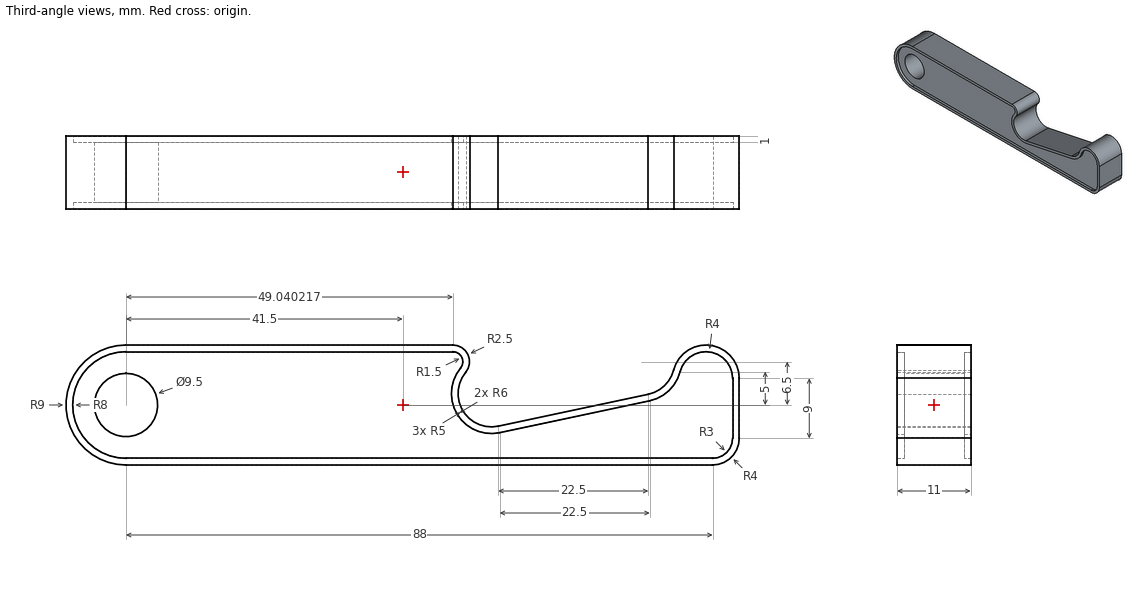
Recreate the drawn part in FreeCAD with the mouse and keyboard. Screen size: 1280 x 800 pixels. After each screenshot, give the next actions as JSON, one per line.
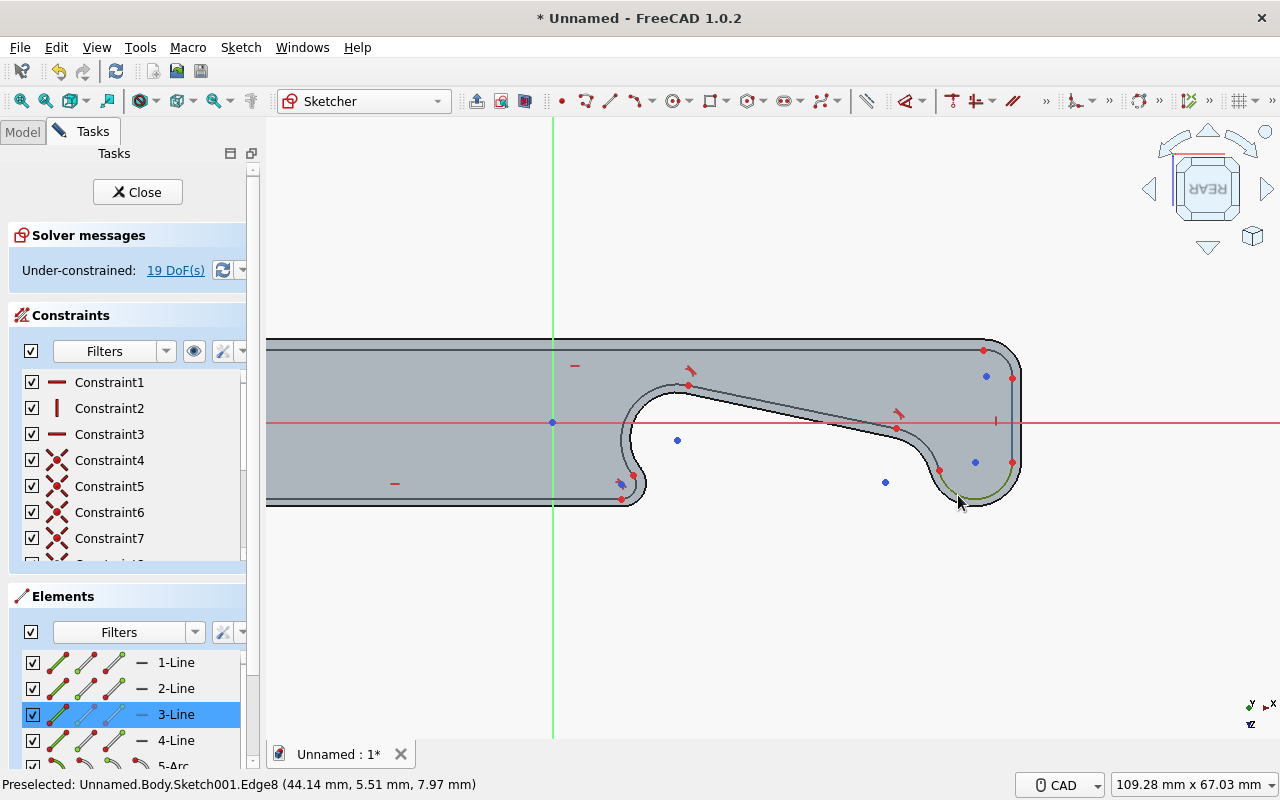
{"action": "key", "text": "t"}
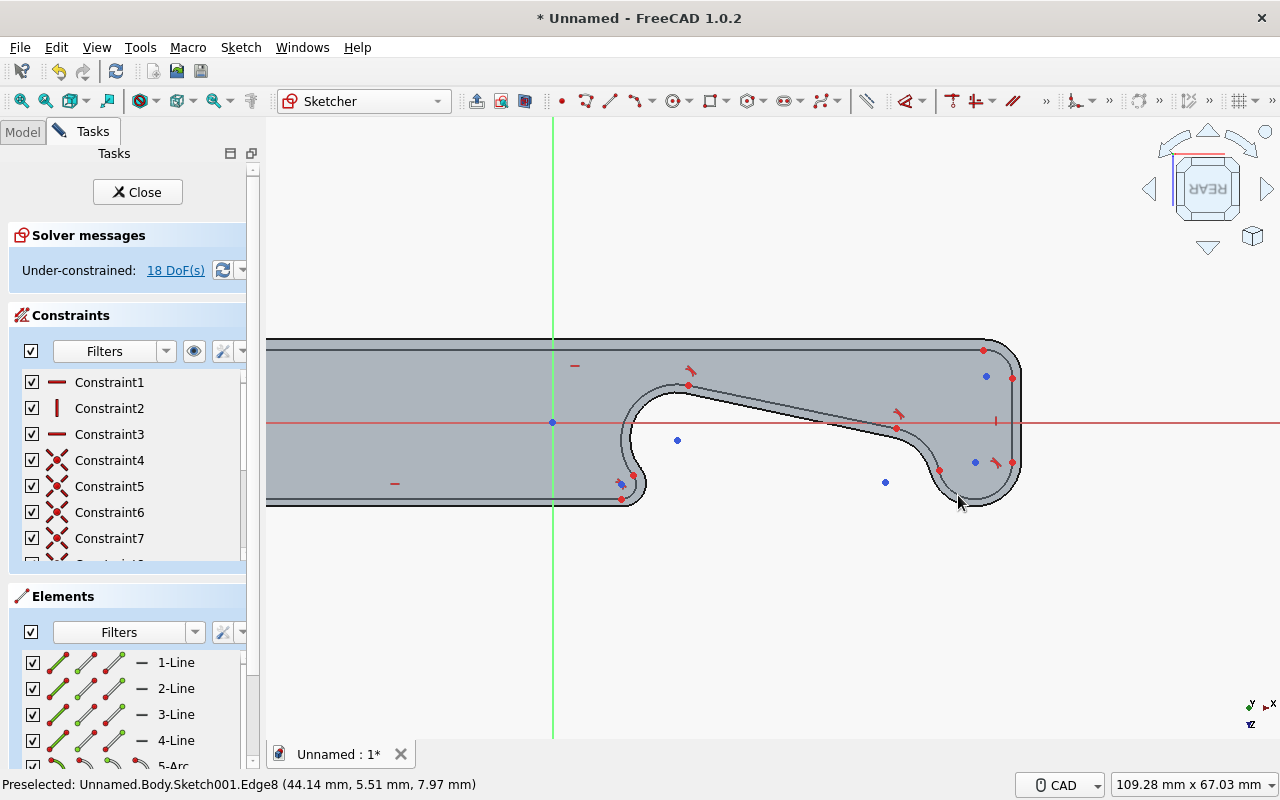
{"action": "left_click", "coordinate": [1012, 437]}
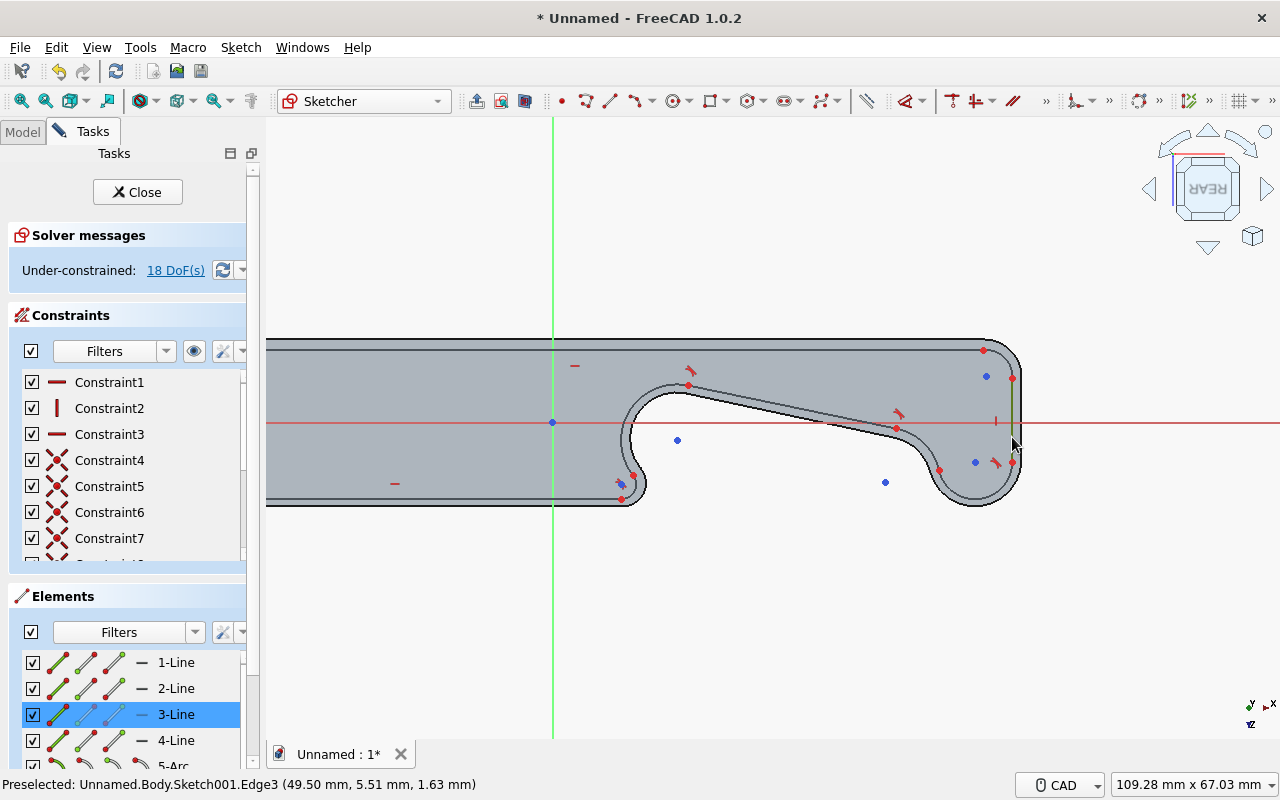
{"action": "left_click", "coordinate": [1010, 365]}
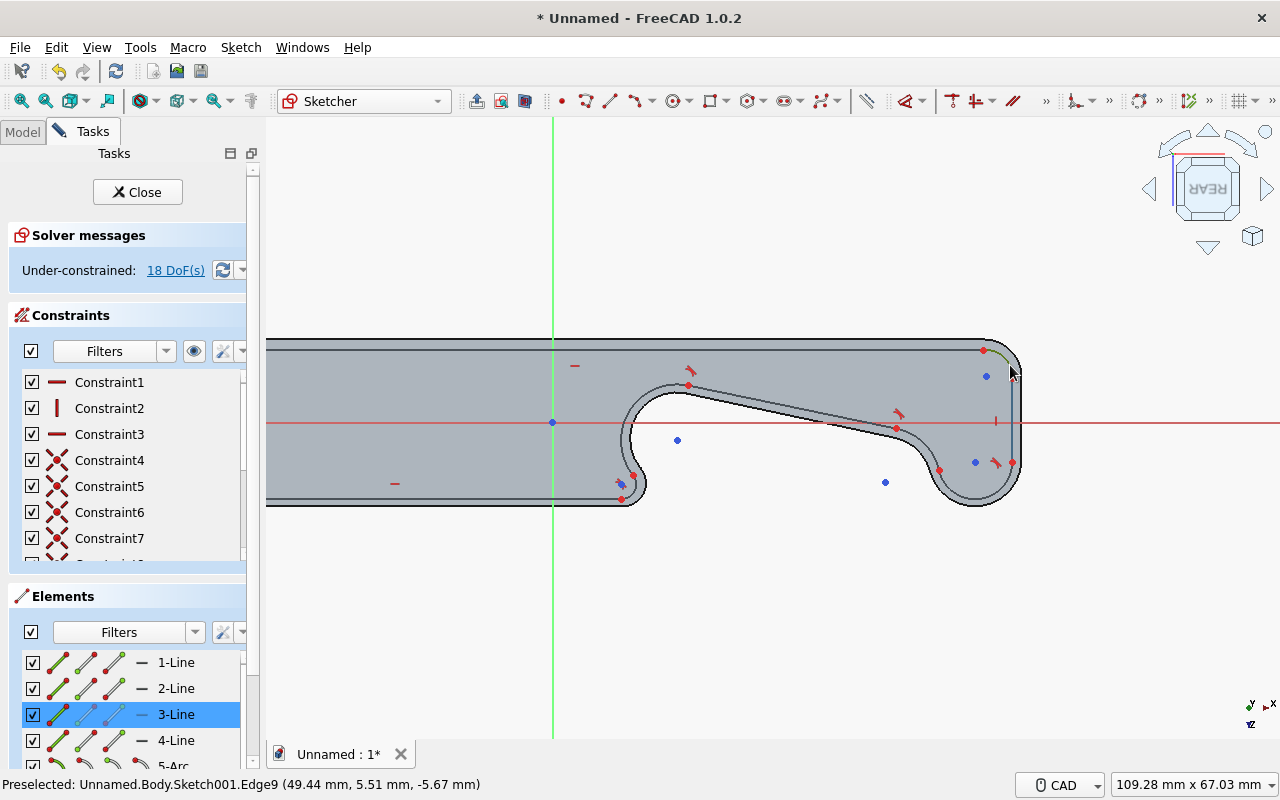
{"action": "key", "text": "t"}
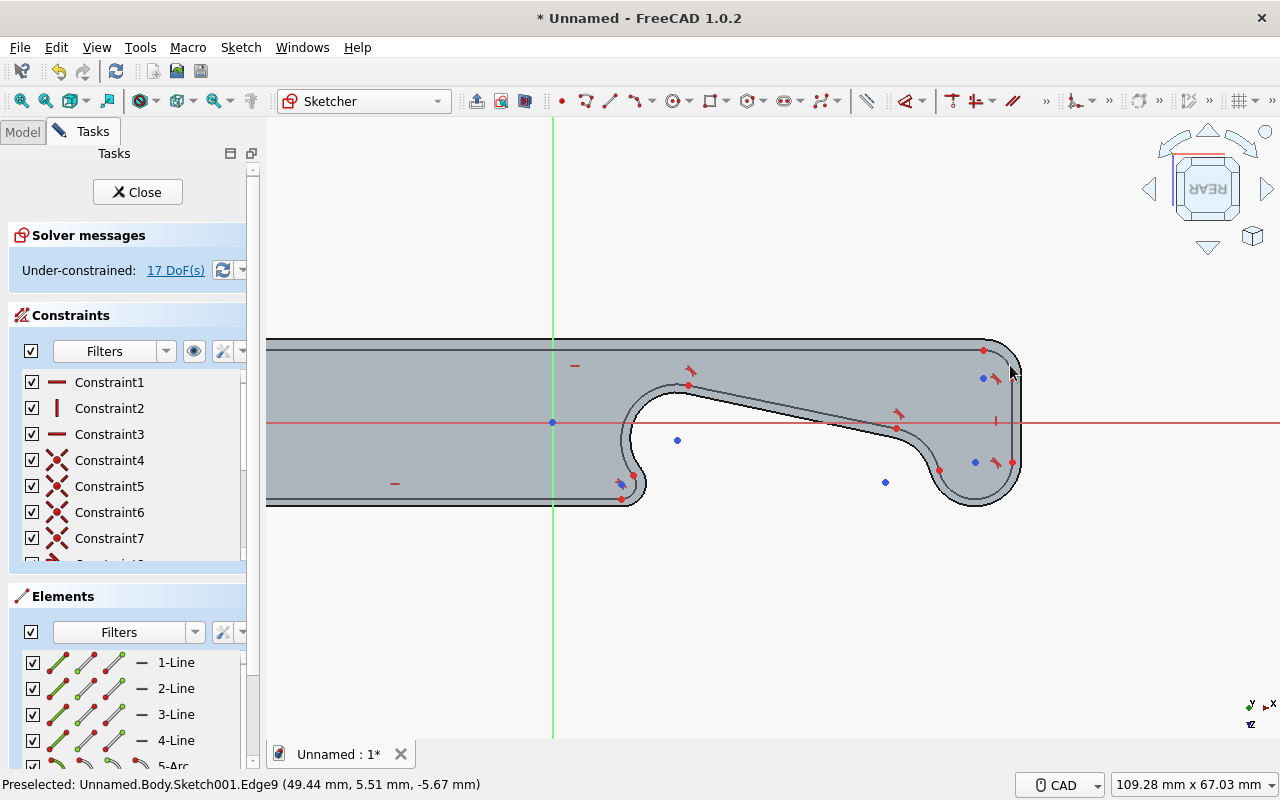
{"action": "left_click", "coordinate": [739, 350]}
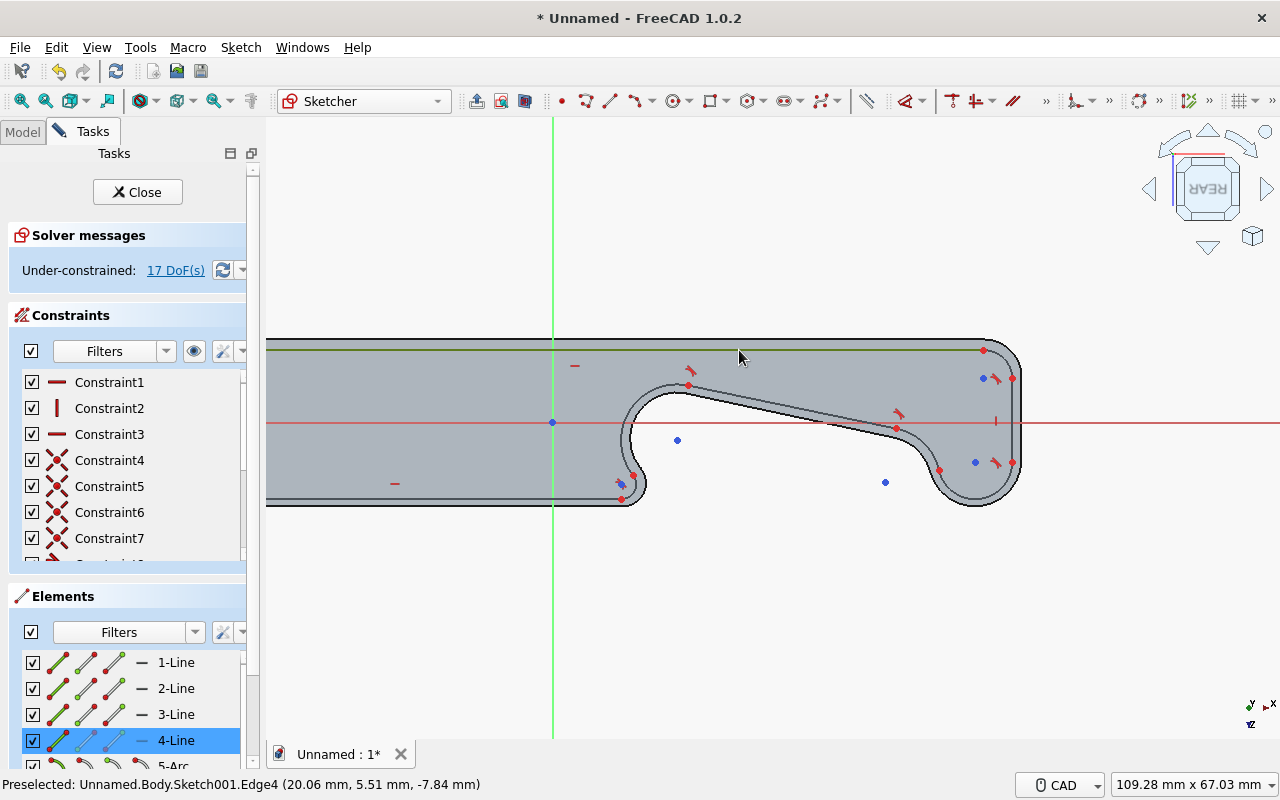
{"action": "left_click", "coordinate": [1009, 366]}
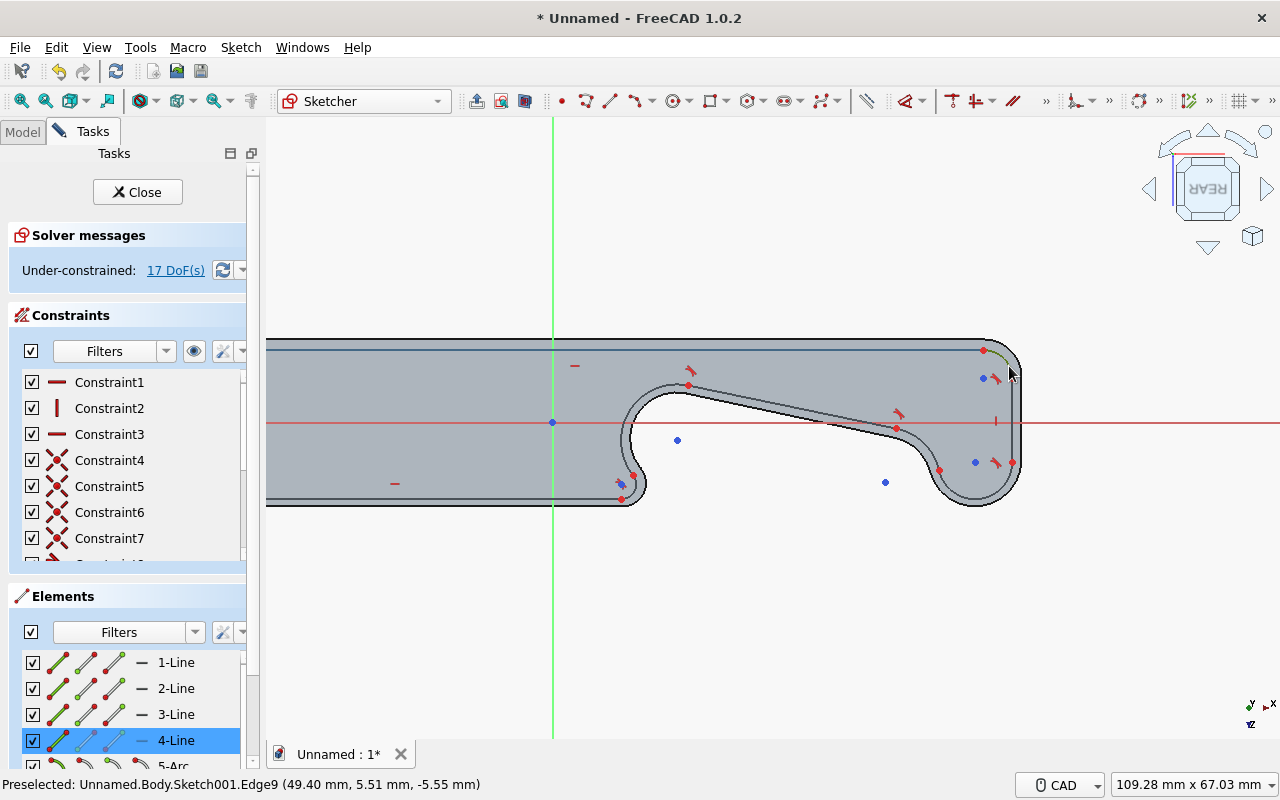
{"action": "key", "text": "t"}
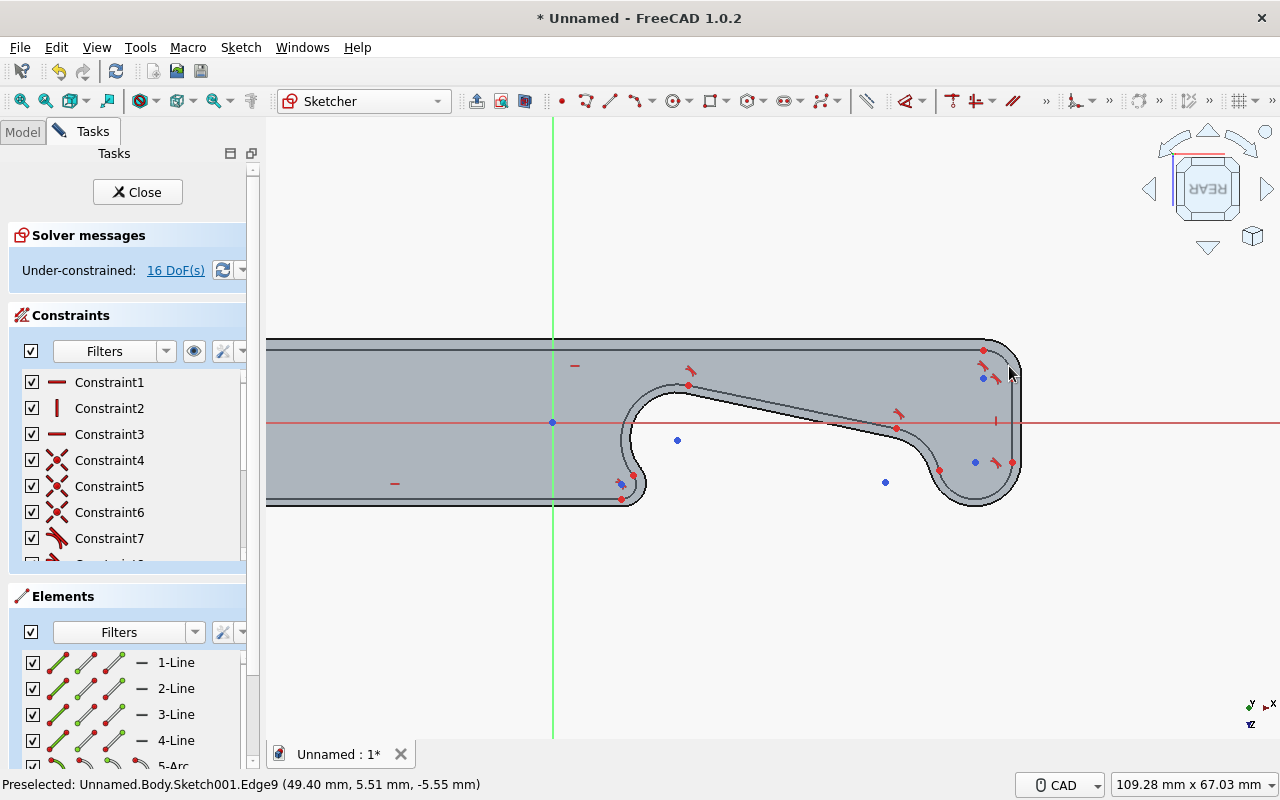
{"action": "left_click", "coordinate": [739, 350]}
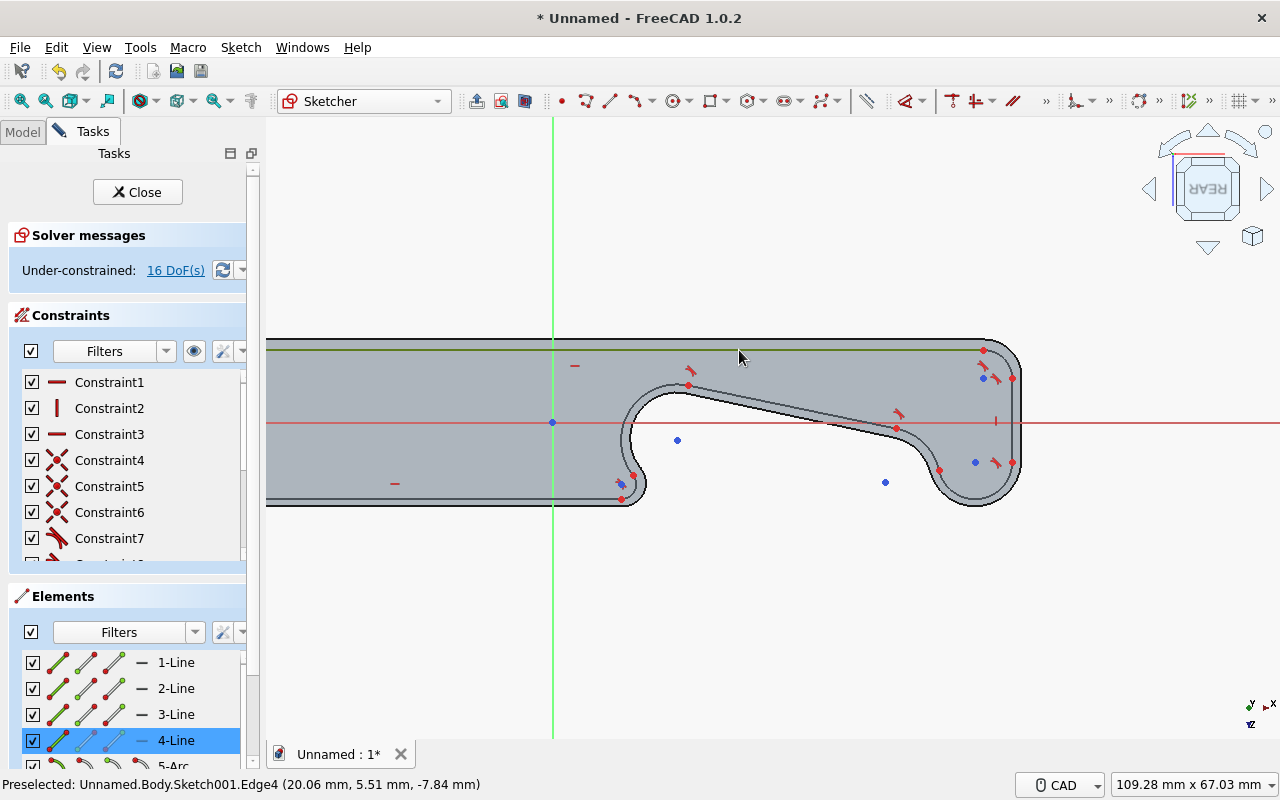
{"action": "scroll", "coordinate": [1013, 438], "scroll_direction": "down", "scroll_amount": 2}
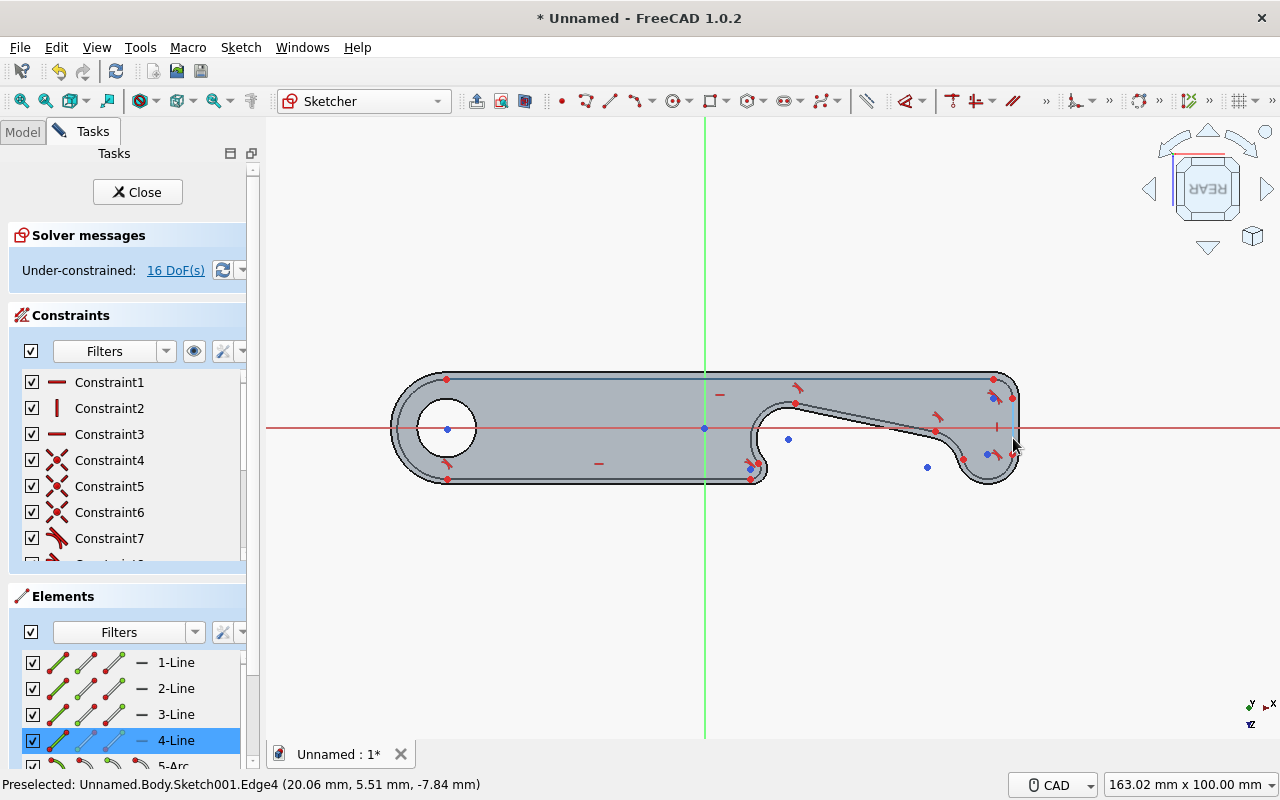
{"action": "left_click", "coordinate": [407, 400]}